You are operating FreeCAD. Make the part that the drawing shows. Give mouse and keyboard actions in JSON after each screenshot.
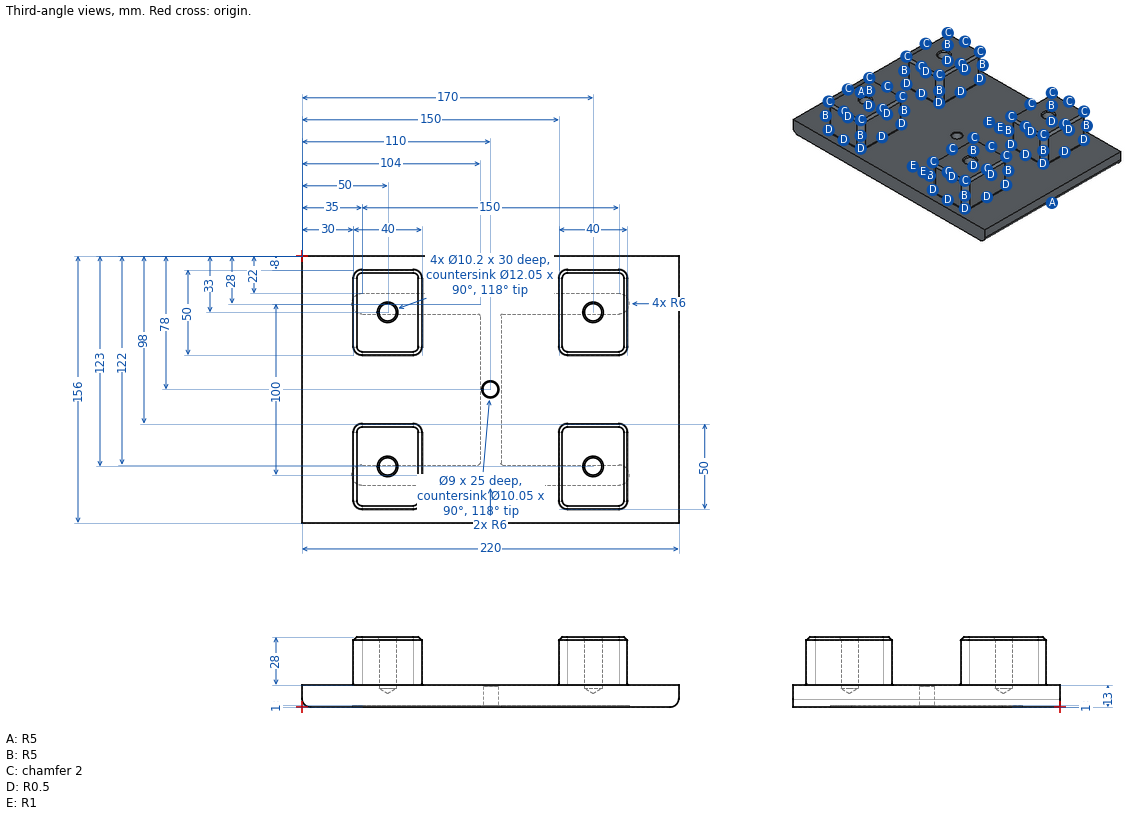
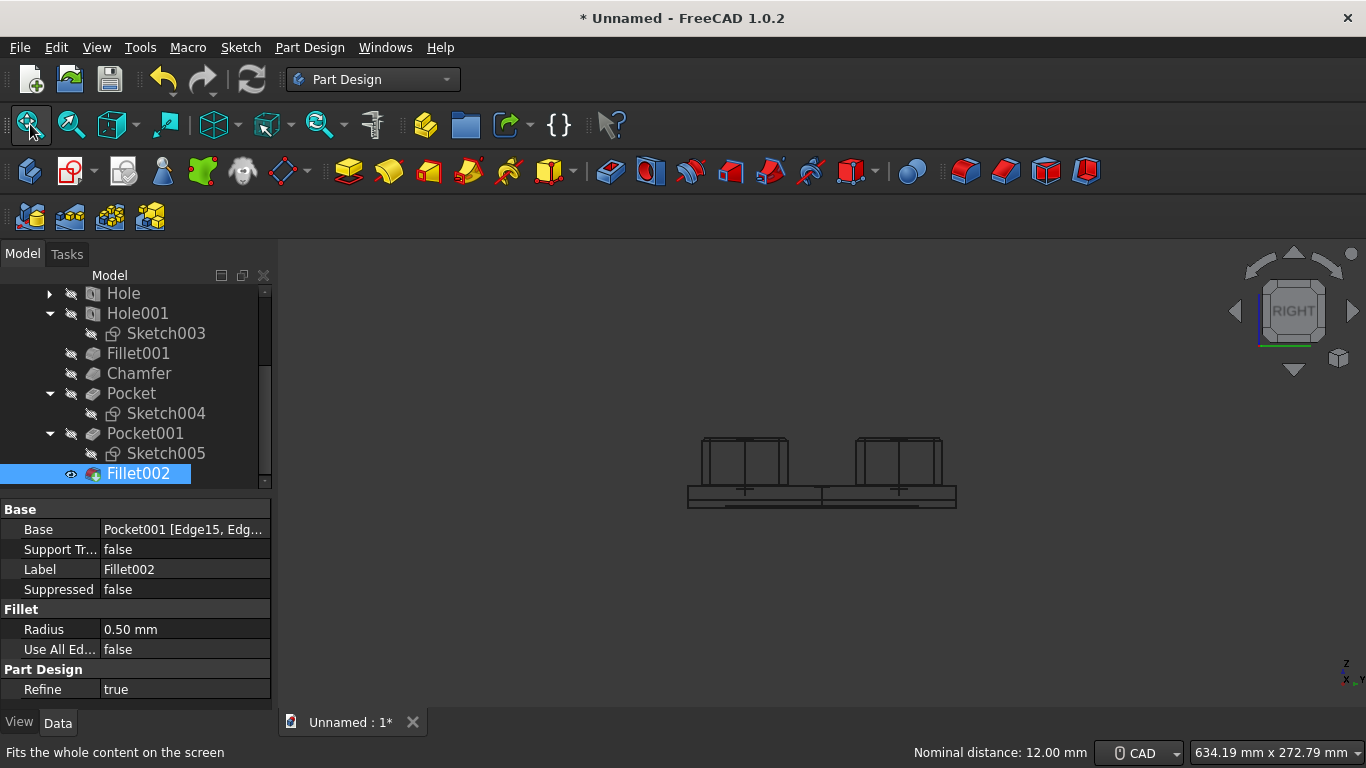
{"action": "scroll", "coordinate": [897, 506], "scroll_direction": "up", "scroll_amount": 15}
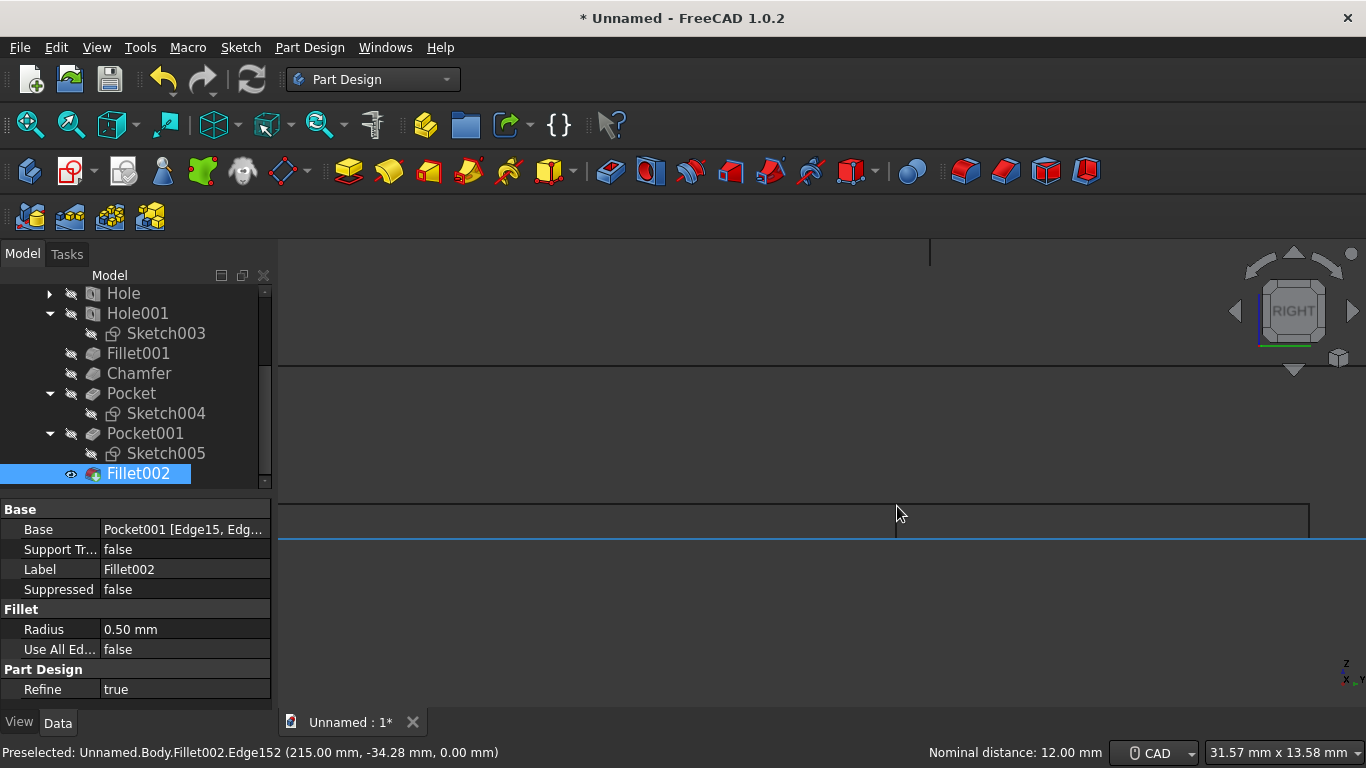
{"action": "key", "text": "v f"}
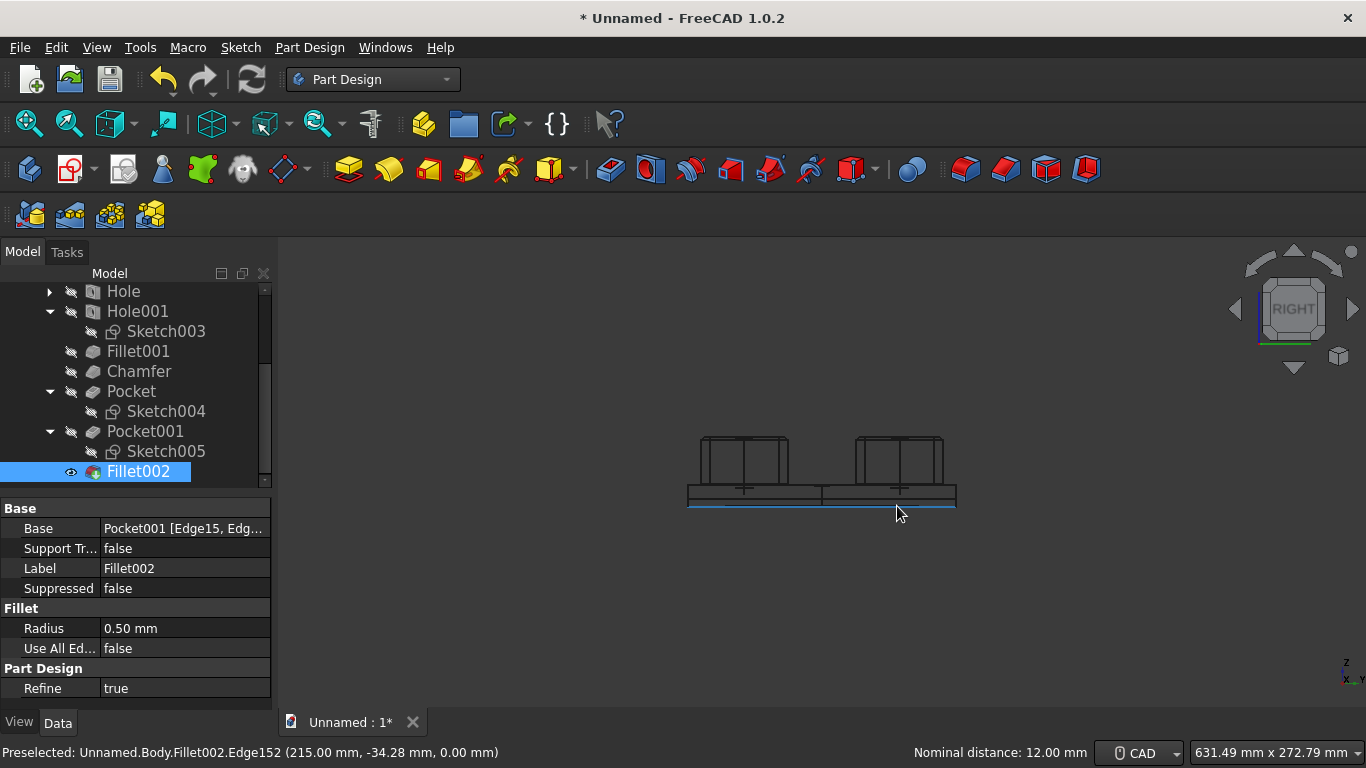
{"action": "key", "text": "5"}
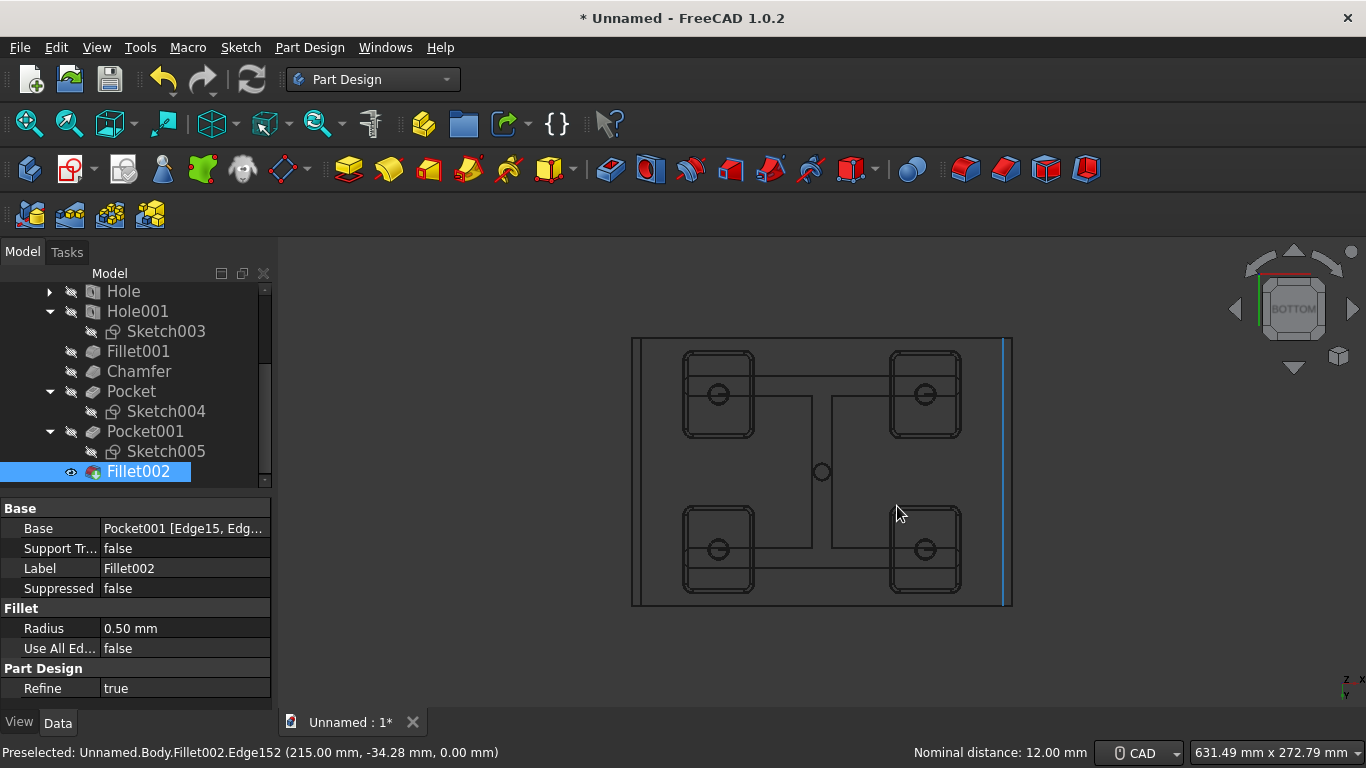
{"action": "scroll", "coordinate": [812, 547], "scroll_direction": "up", "scroll_amount": 15}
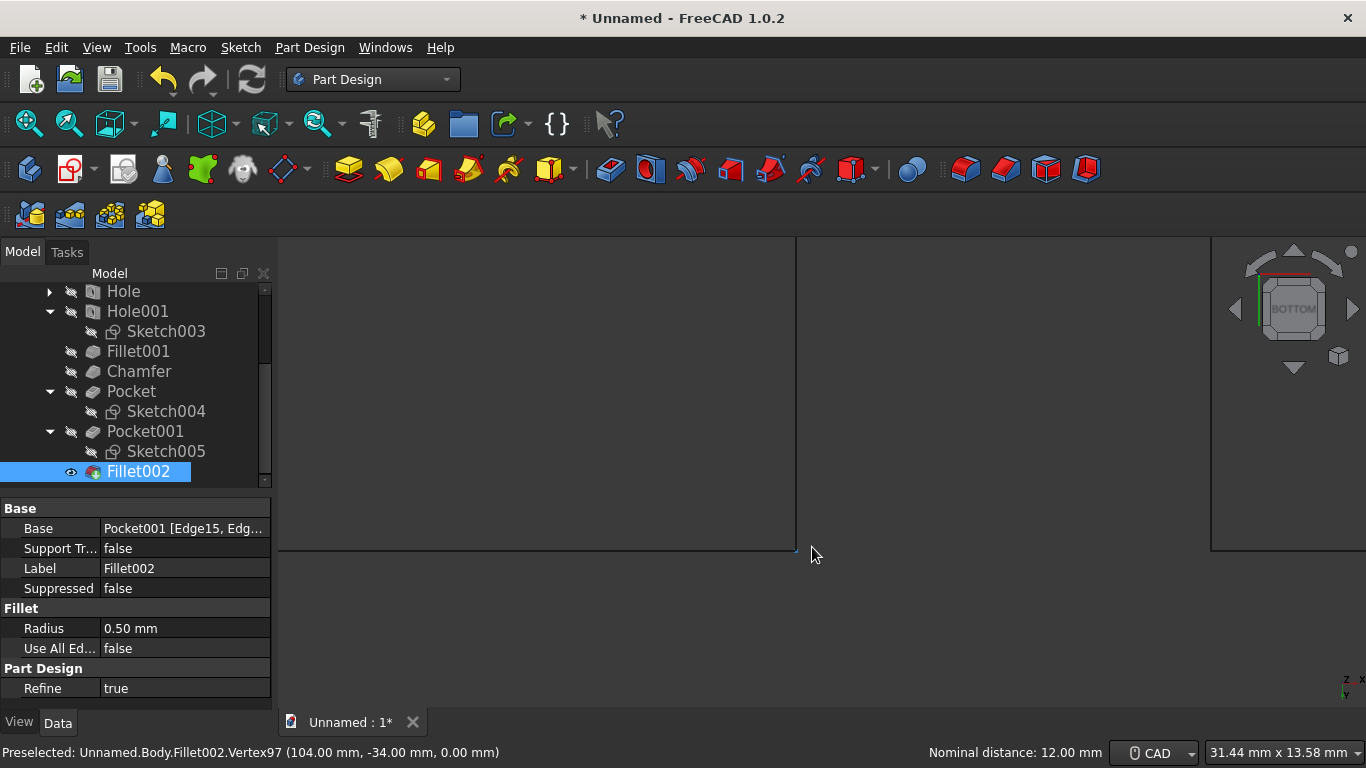
{"action": "key", "text": "v f"}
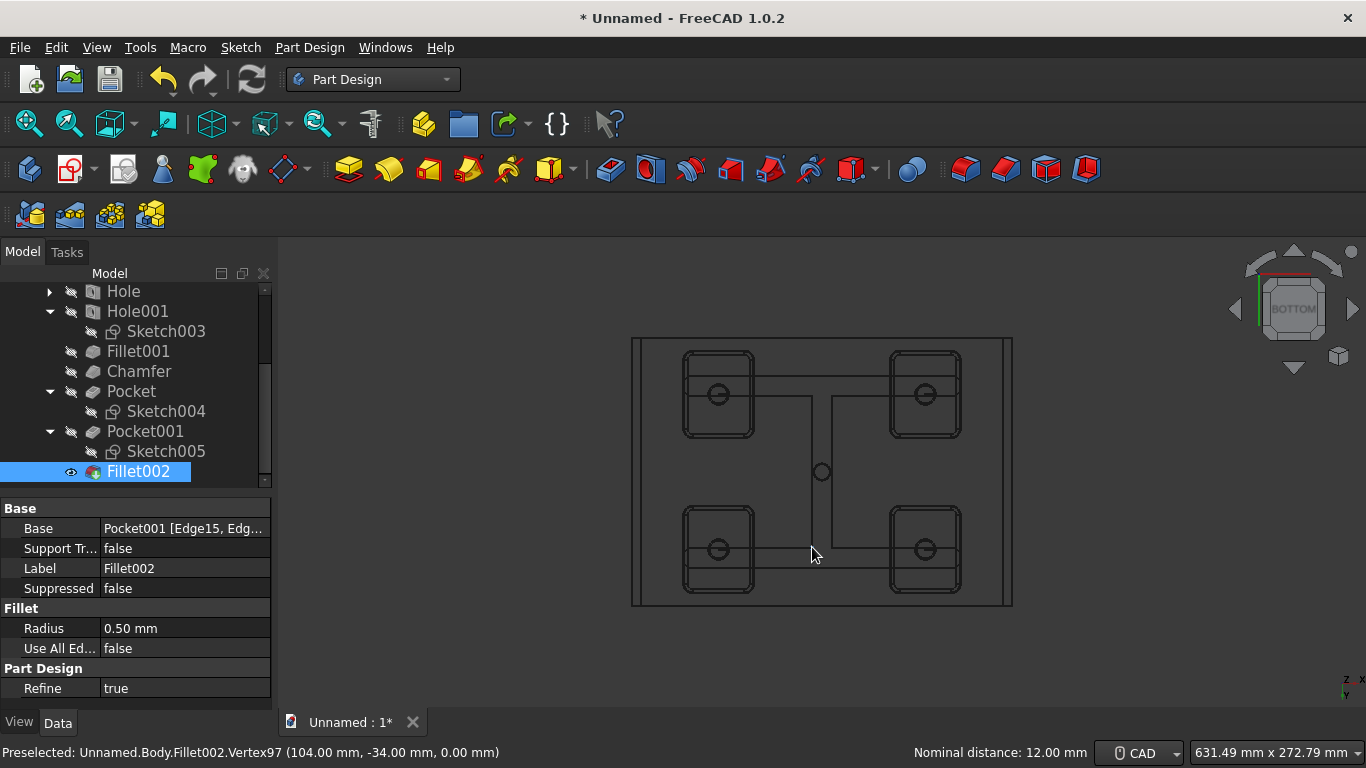
{"action": "key", "text": "4"}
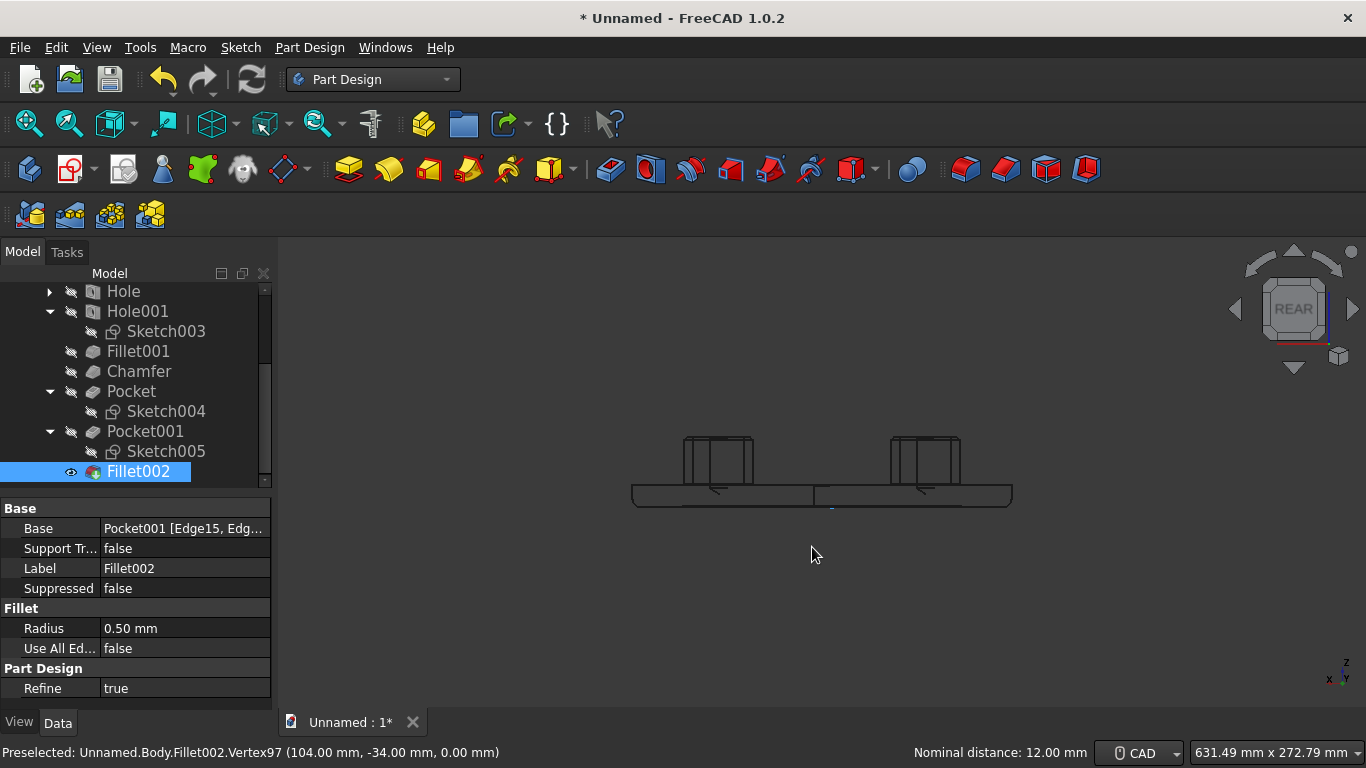
{"action": "key", "text": "v f"}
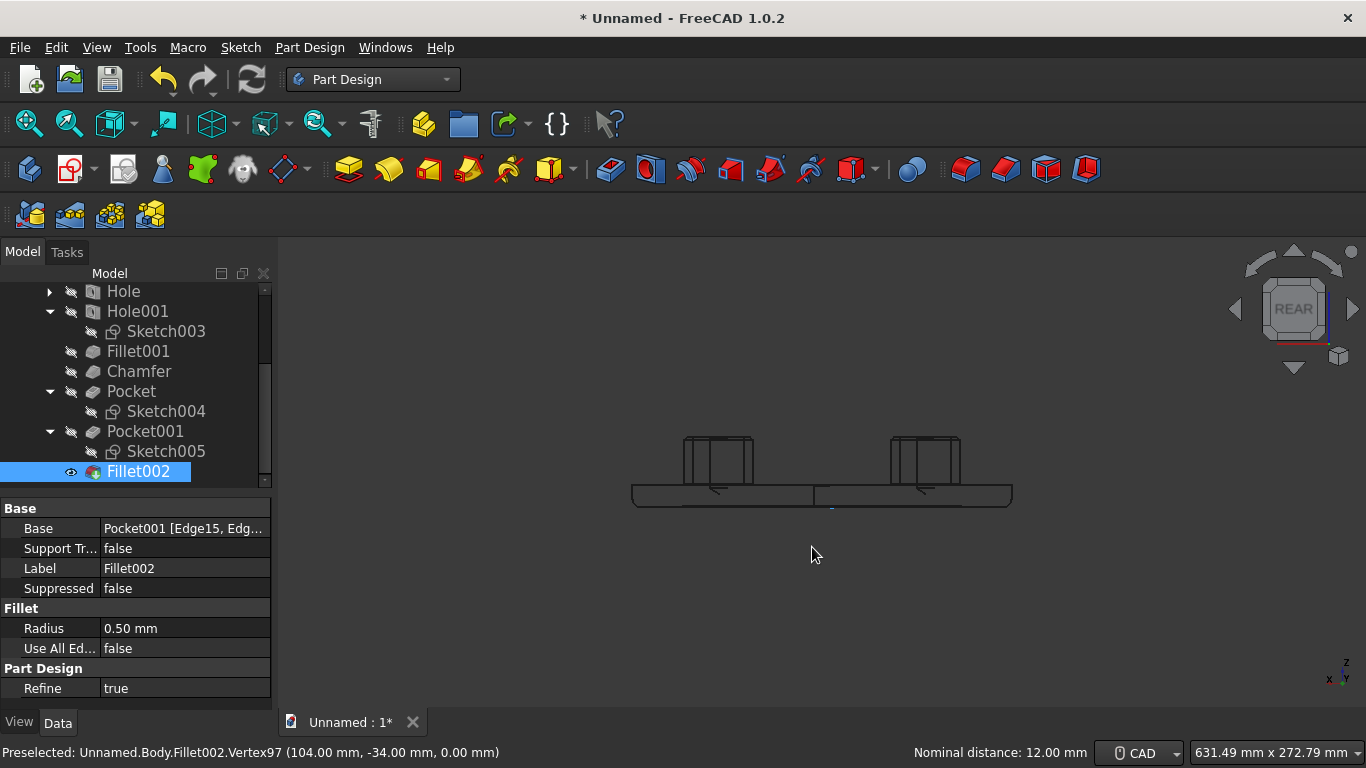
{"action": "scroll", "coordinate": [832, 505], "scroll_direction": "up", "scroll_amount": 15}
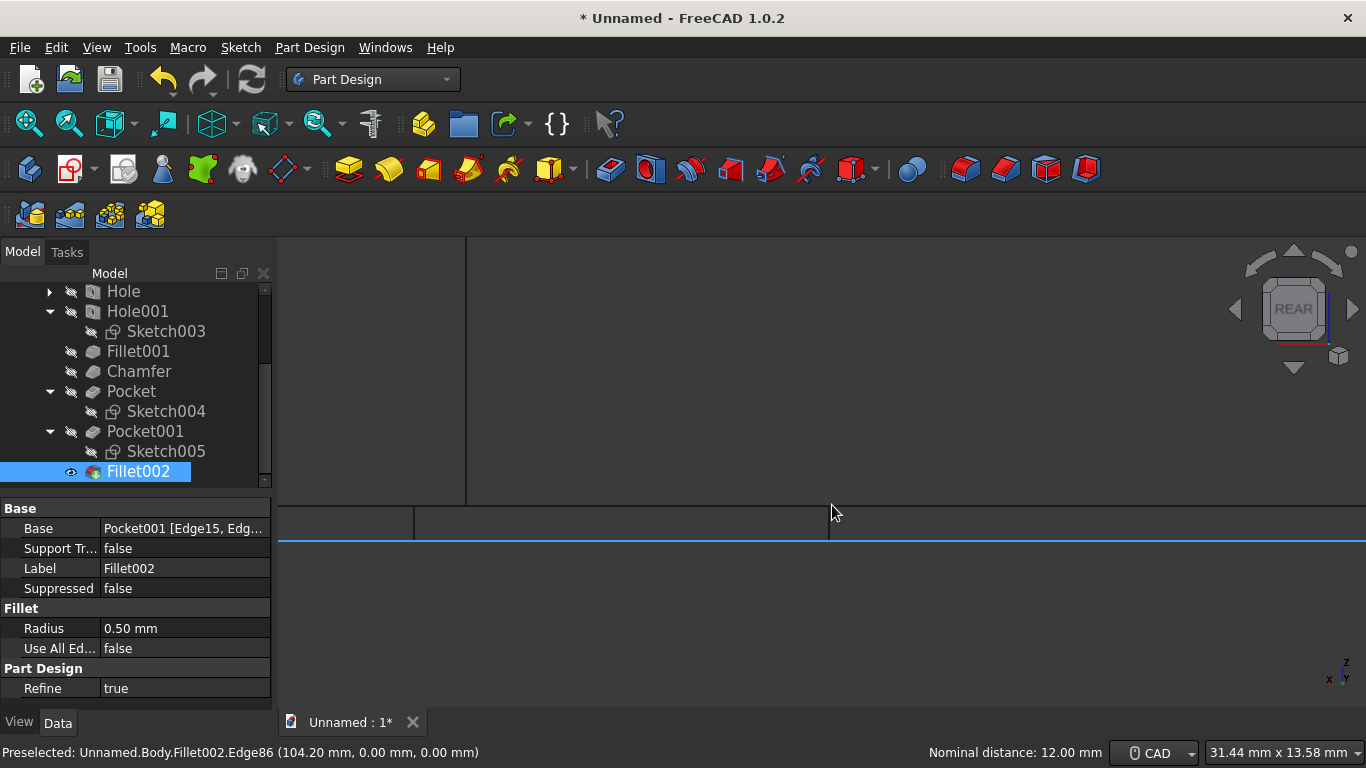
{"action": "left_click", "coordinate": [829, 522], "text": "ctrl"}